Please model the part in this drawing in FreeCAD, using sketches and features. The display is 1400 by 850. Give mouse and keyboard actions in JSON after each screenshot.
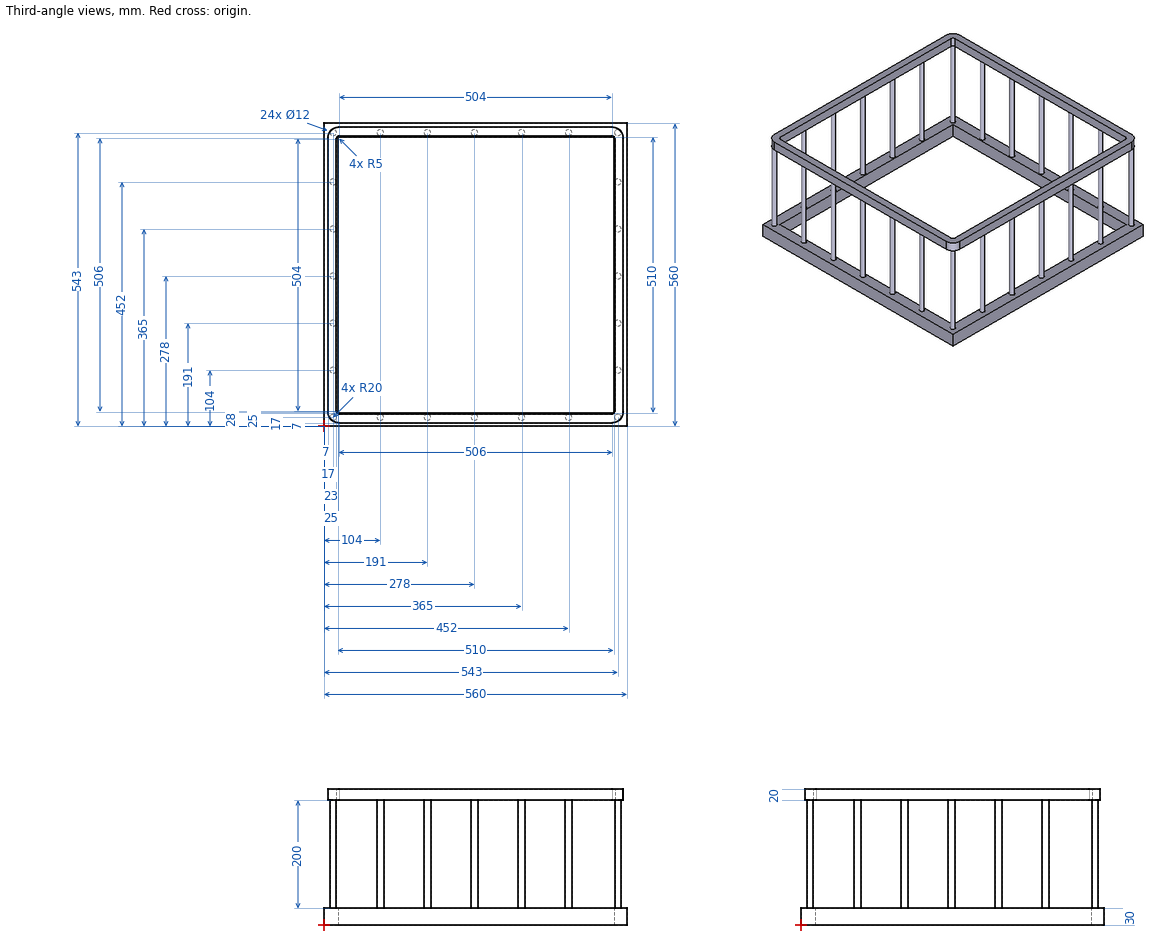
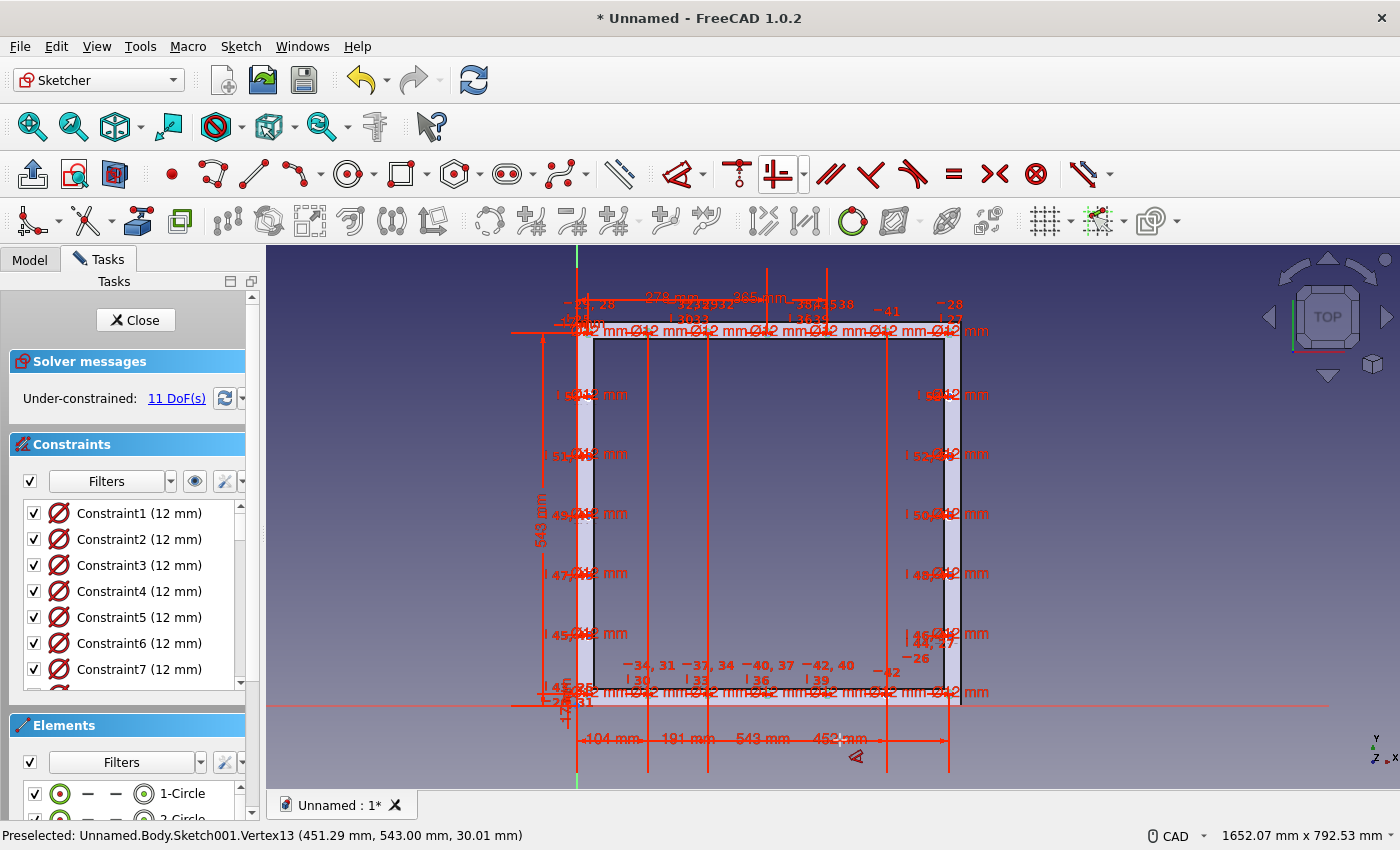
{"action": "left_click", "coordinate": [887, 694]}
{"action": "left_click", "coordinate": [732, 660]}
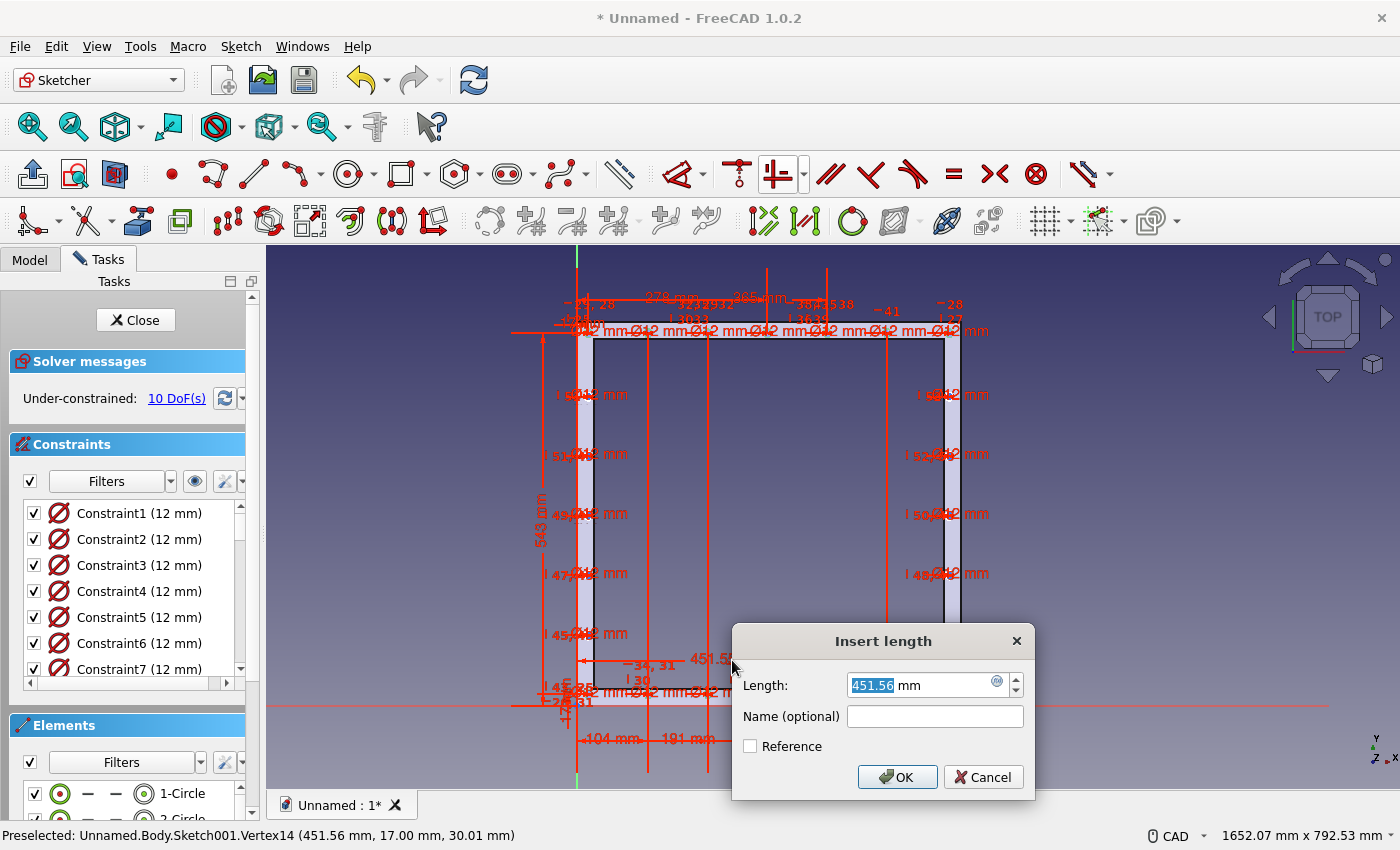
{"action": "type", "text": "452"}
{"action": "key", "text": "Return"}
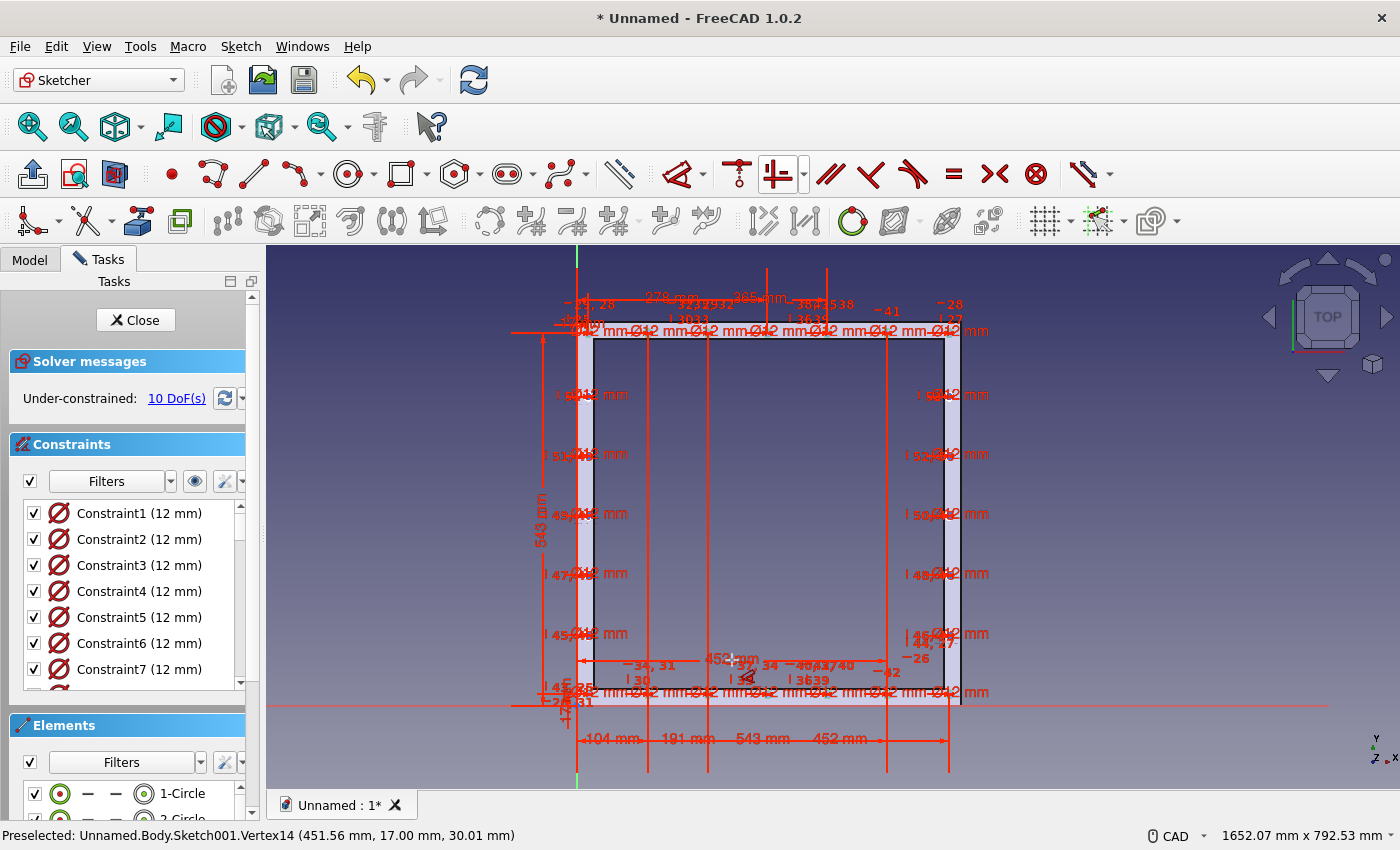
{"action": "left_click", "coordinate": [588, 635]}
{"action": "left_click", "coordinate": [543, 671]}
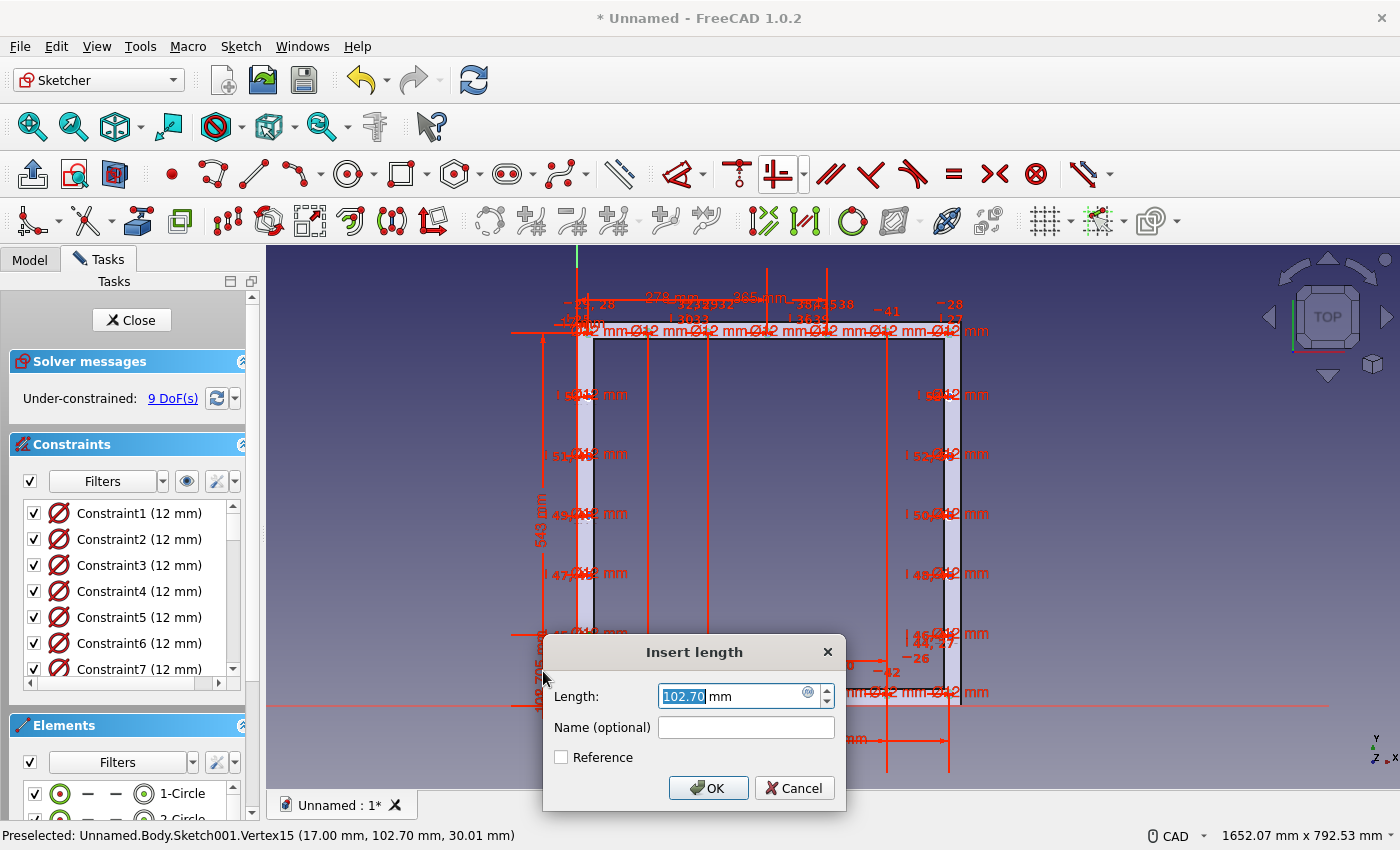
{"action": "type", "text": "104"}
{"action": "key", "text": "Return"}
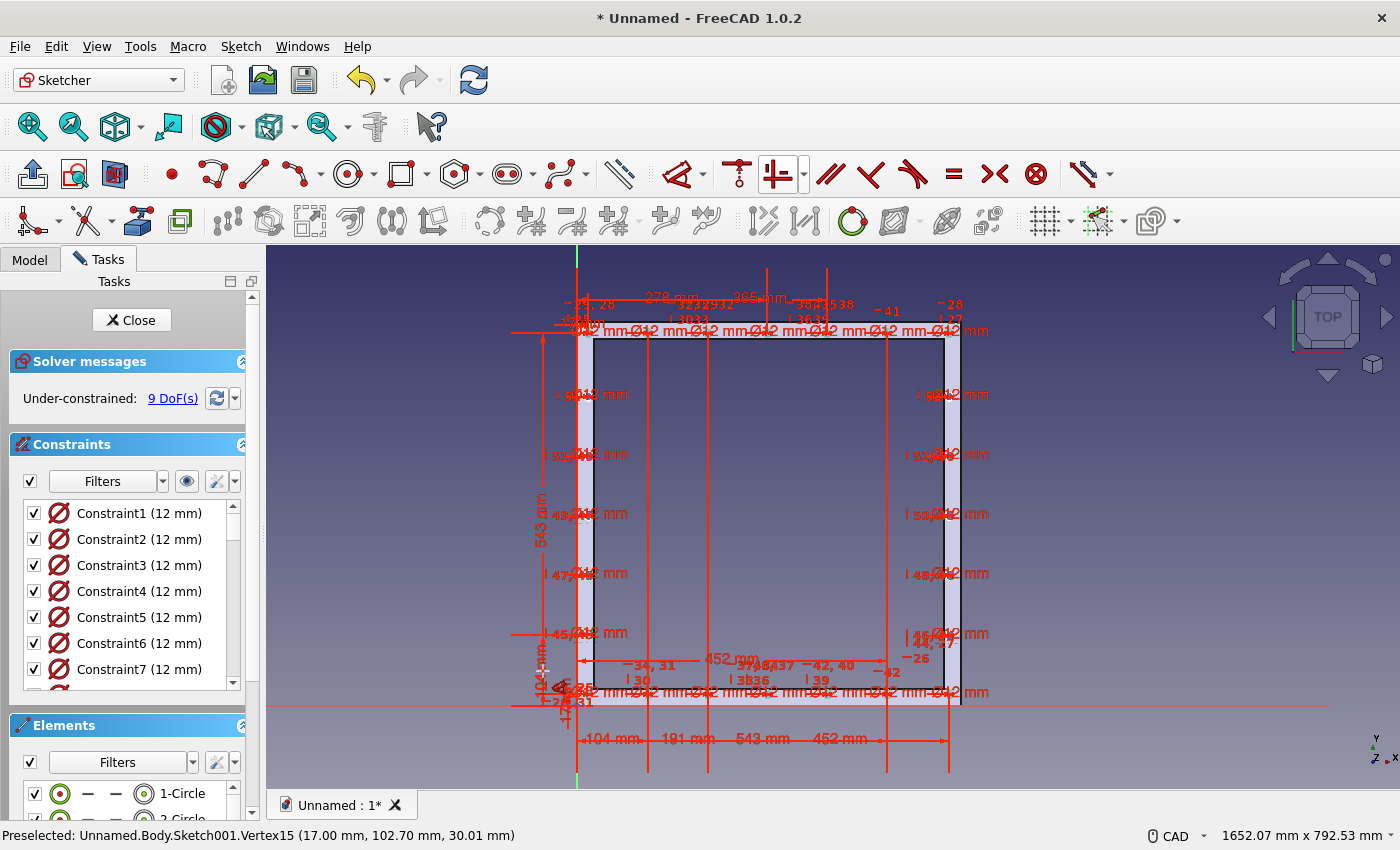
{"action": "left_click", "coordinate": [949, 636]}
{"action": "left_click", "coordinate": [543, 646]}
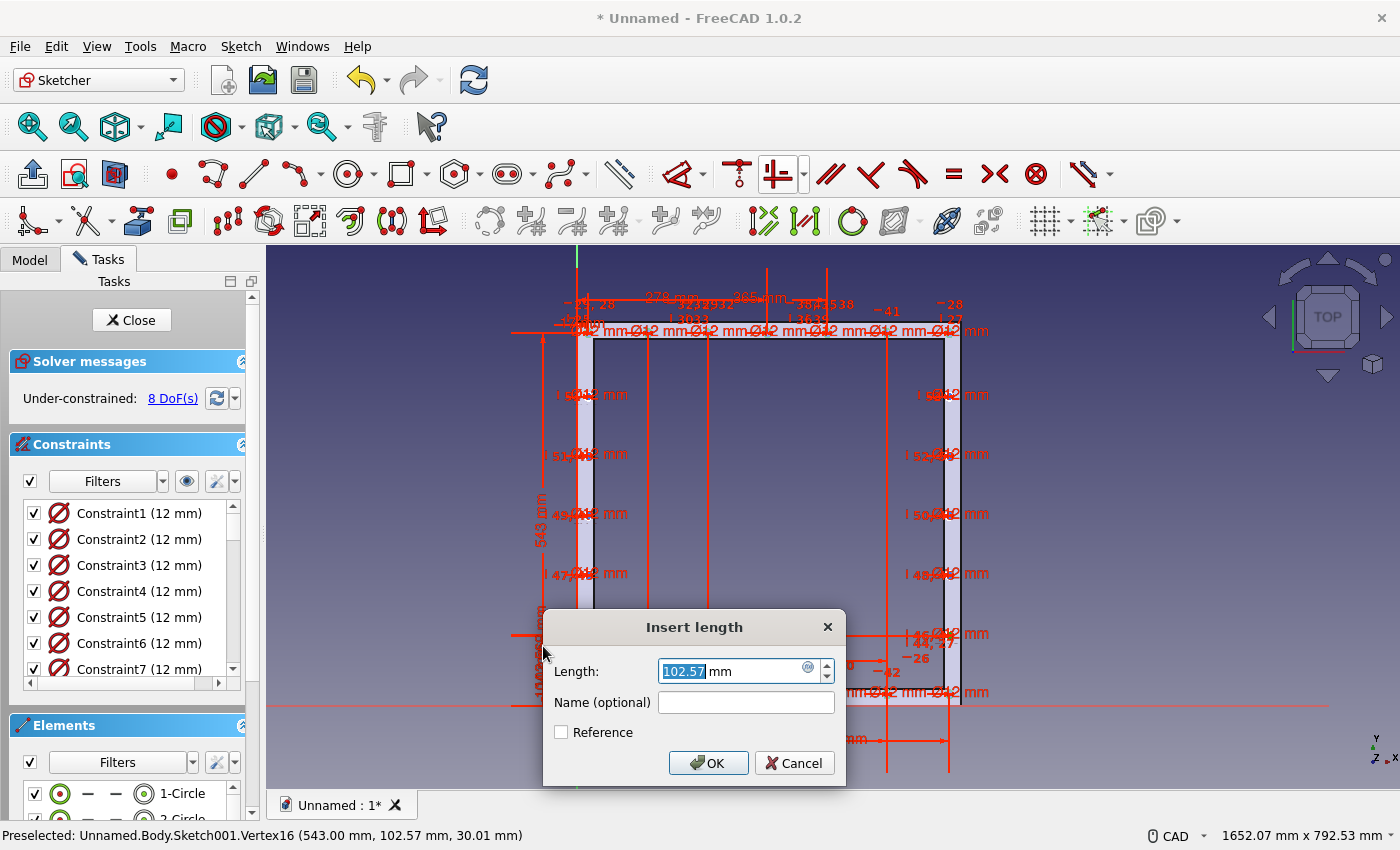
{"action": "type", "text": "104"}
{"action": "key", "text": "Return"}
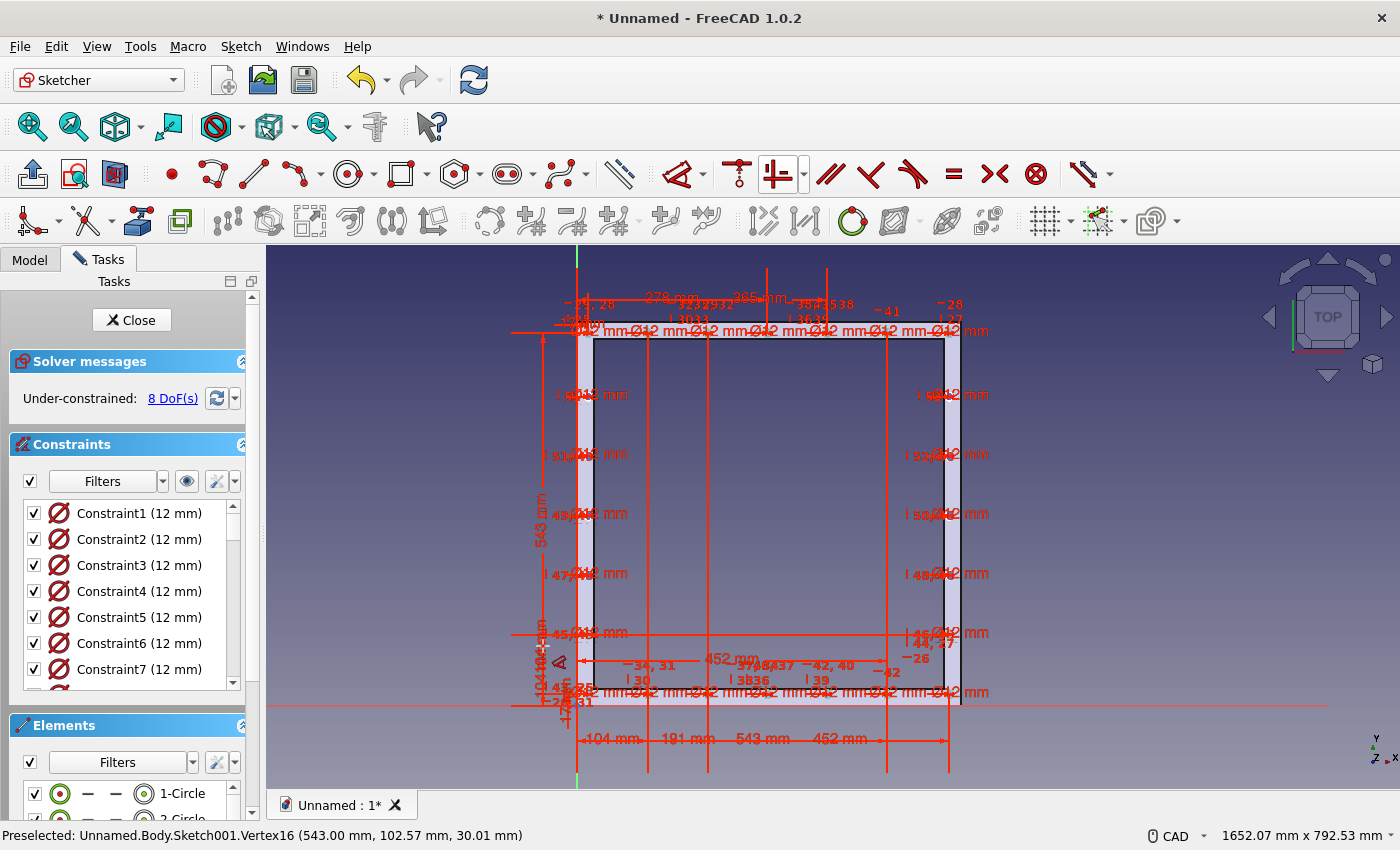
{"action": "left_click", "coordinate": [588, 575]}
{"action": "left_click", "coordinate": [543, 611]}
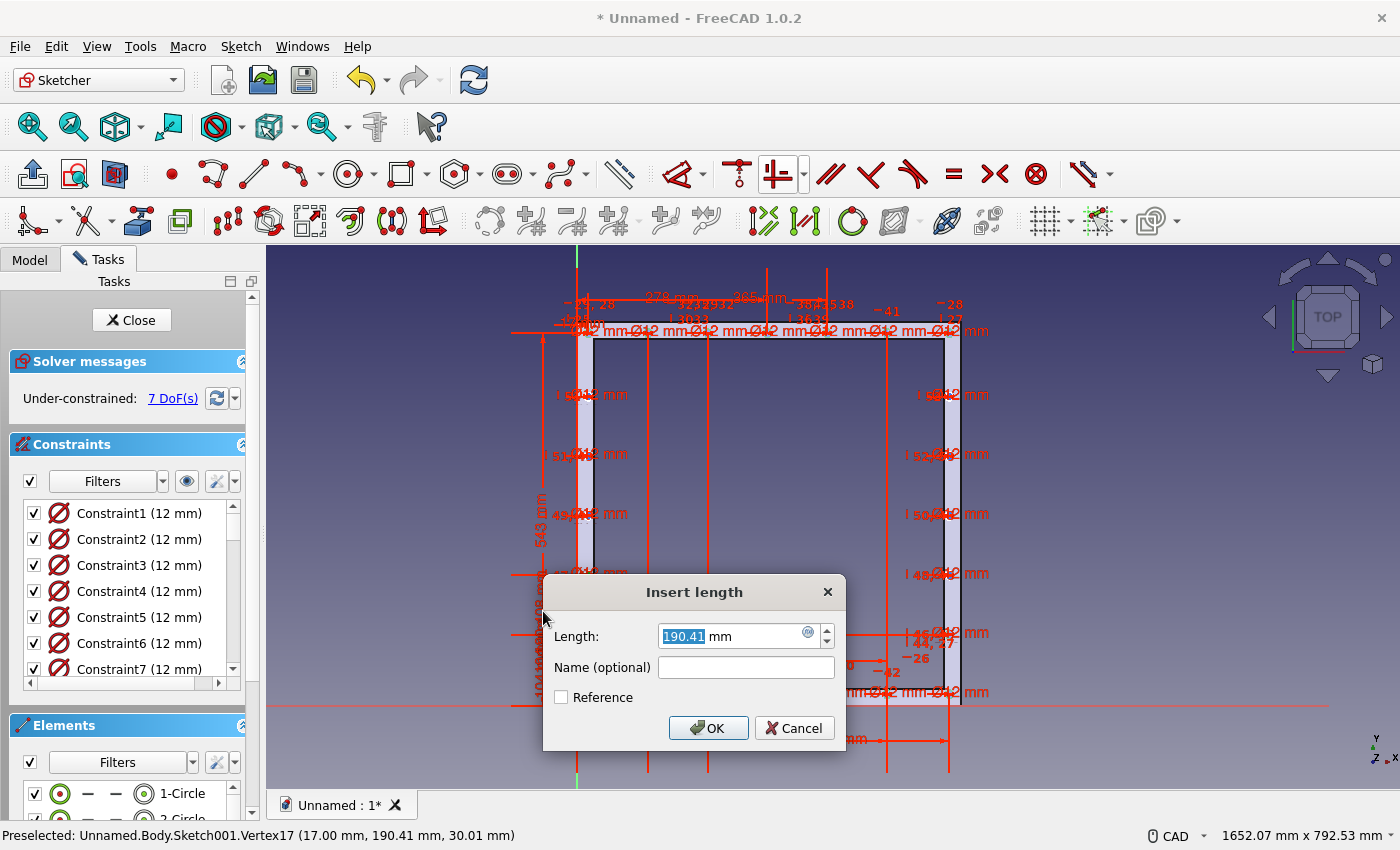
{"action": "type", "text": "191"}
{"action": "key", "text": "Return"}